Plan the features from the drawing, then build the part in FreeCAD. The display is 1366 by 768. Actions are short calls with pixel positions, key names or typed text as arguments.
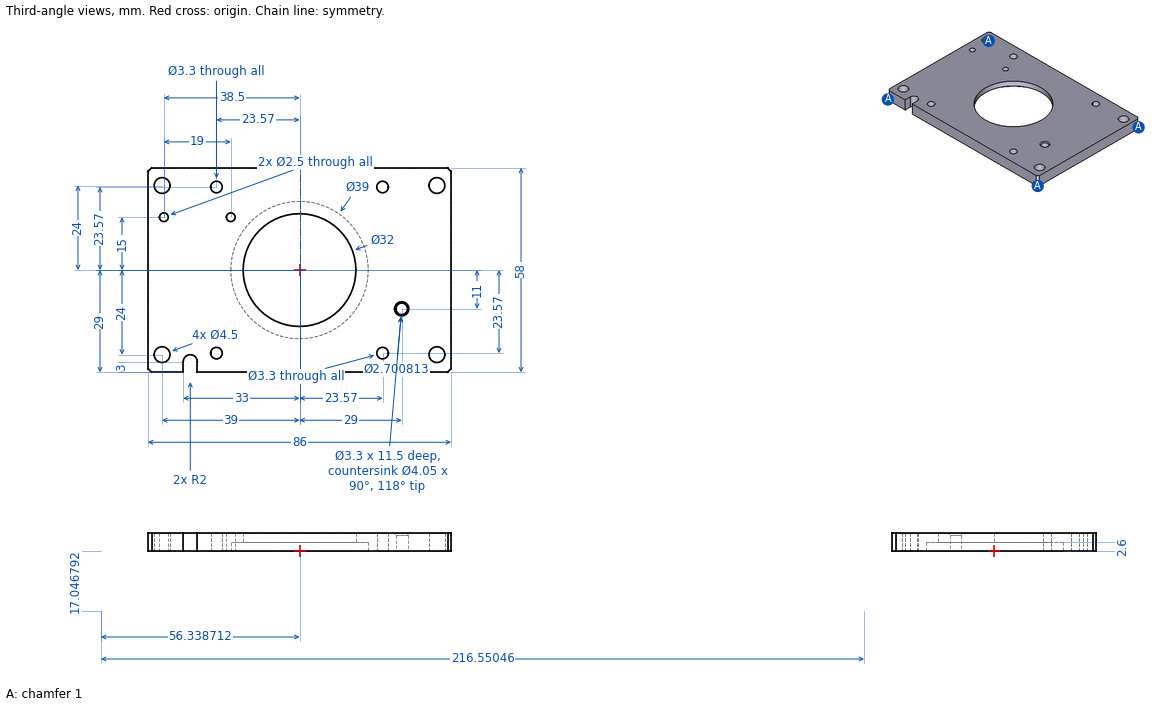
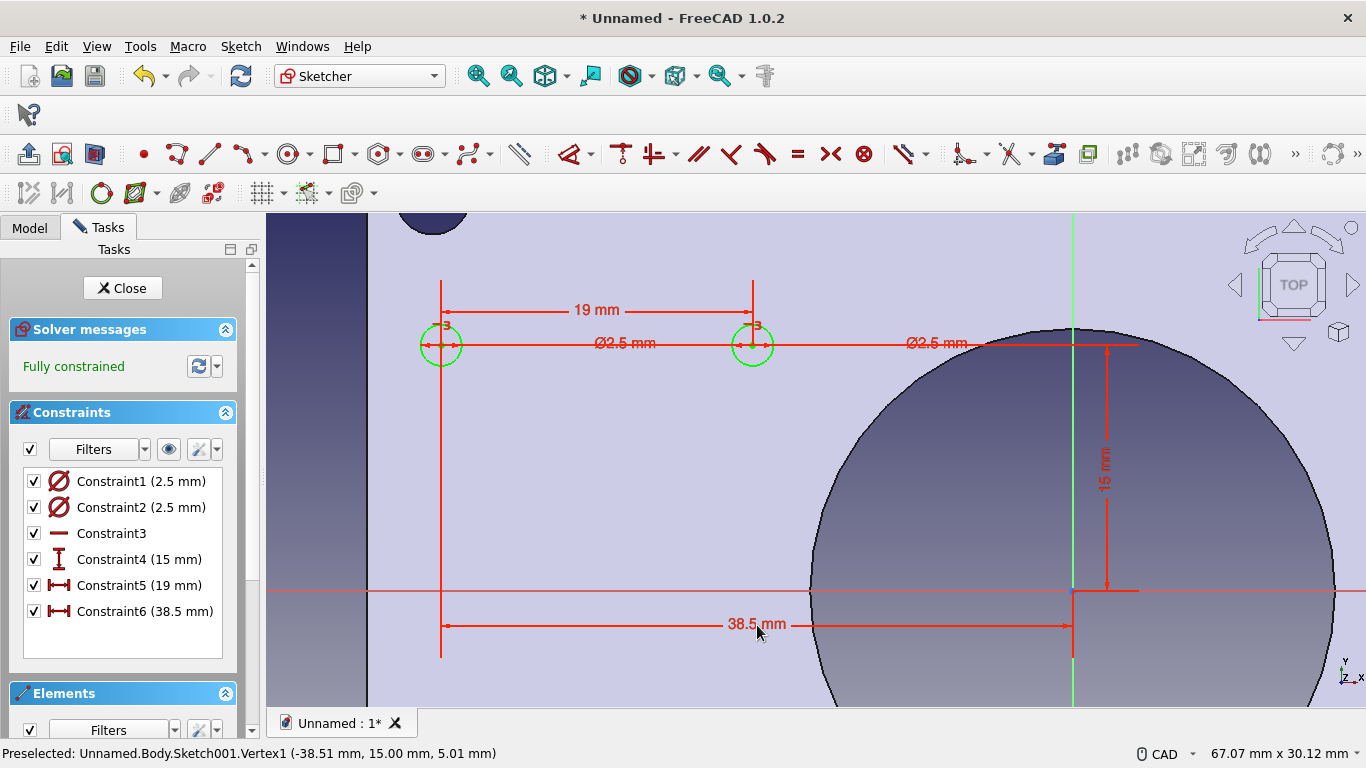
click(123, 288)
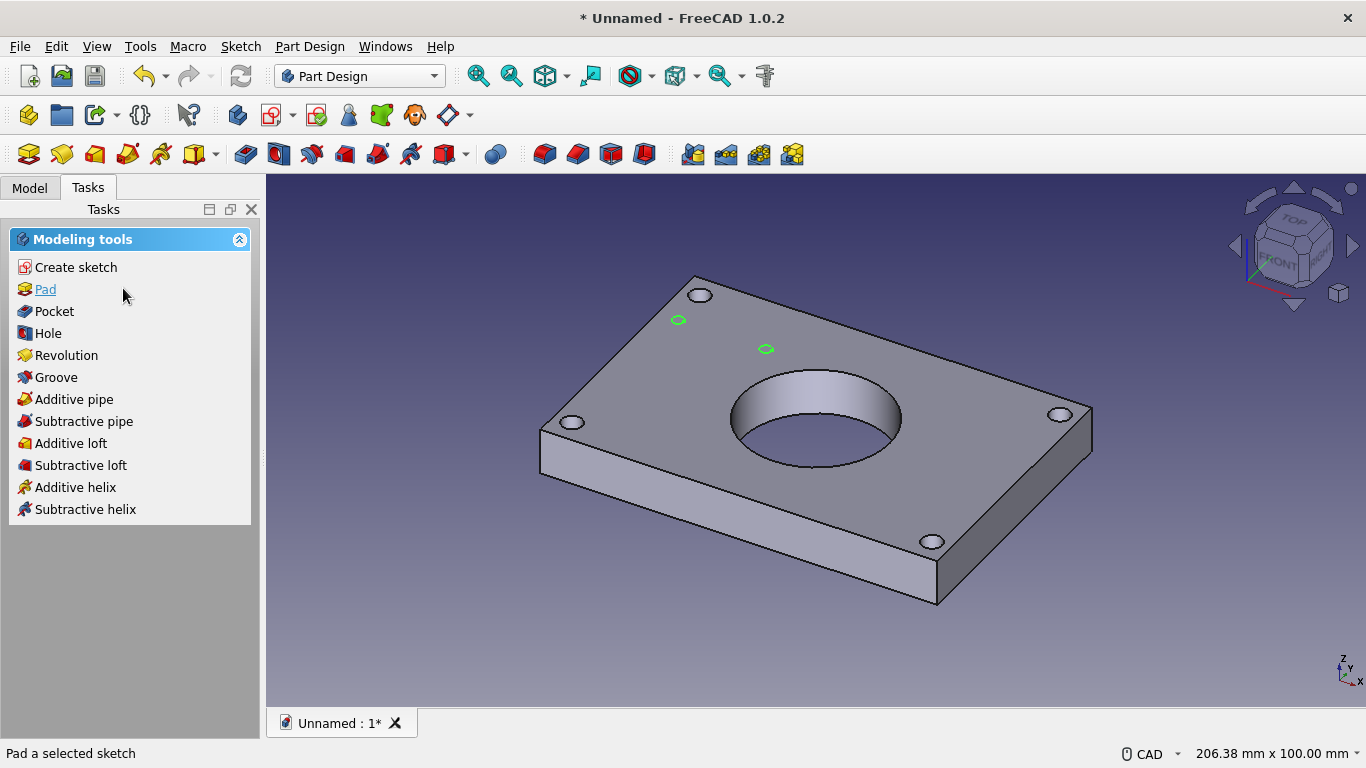
click(279, 154)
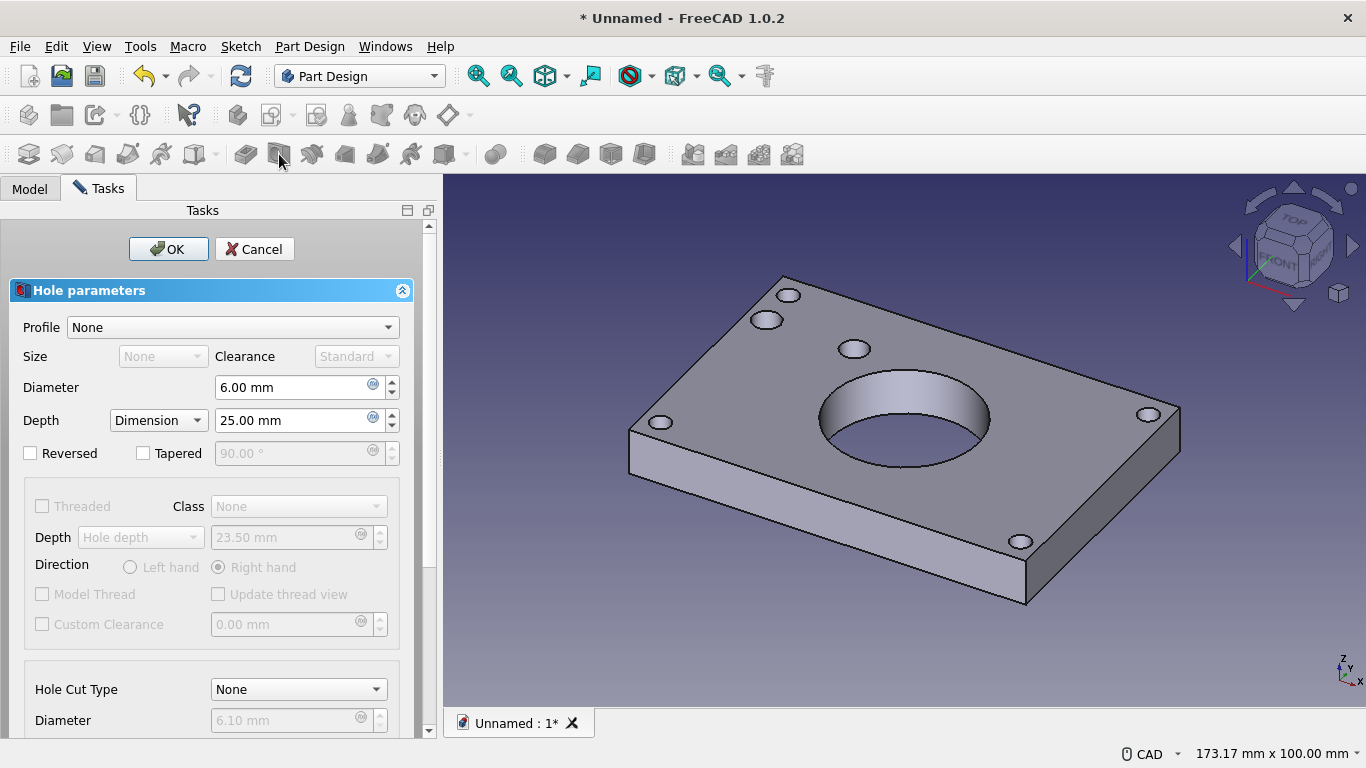
triple_click(300, 388)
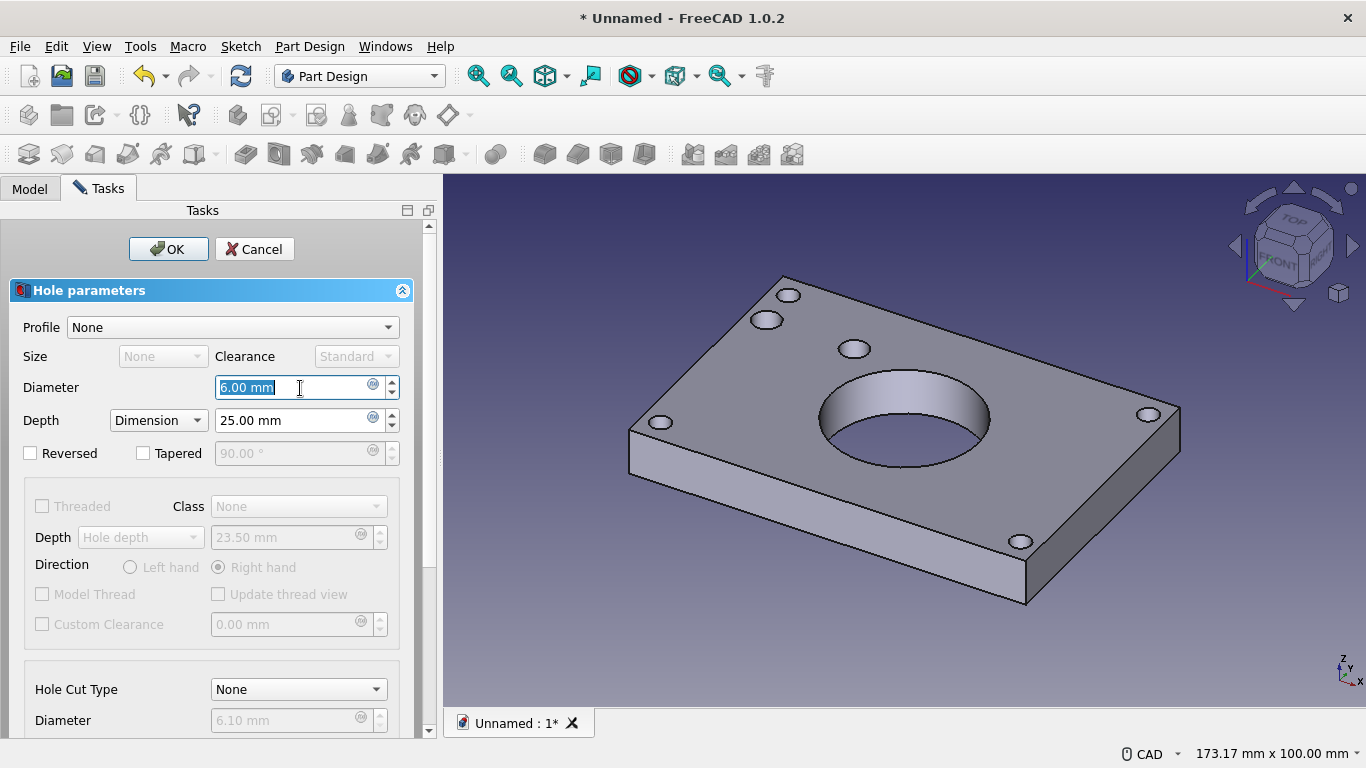
text(2.5)
key(Tab)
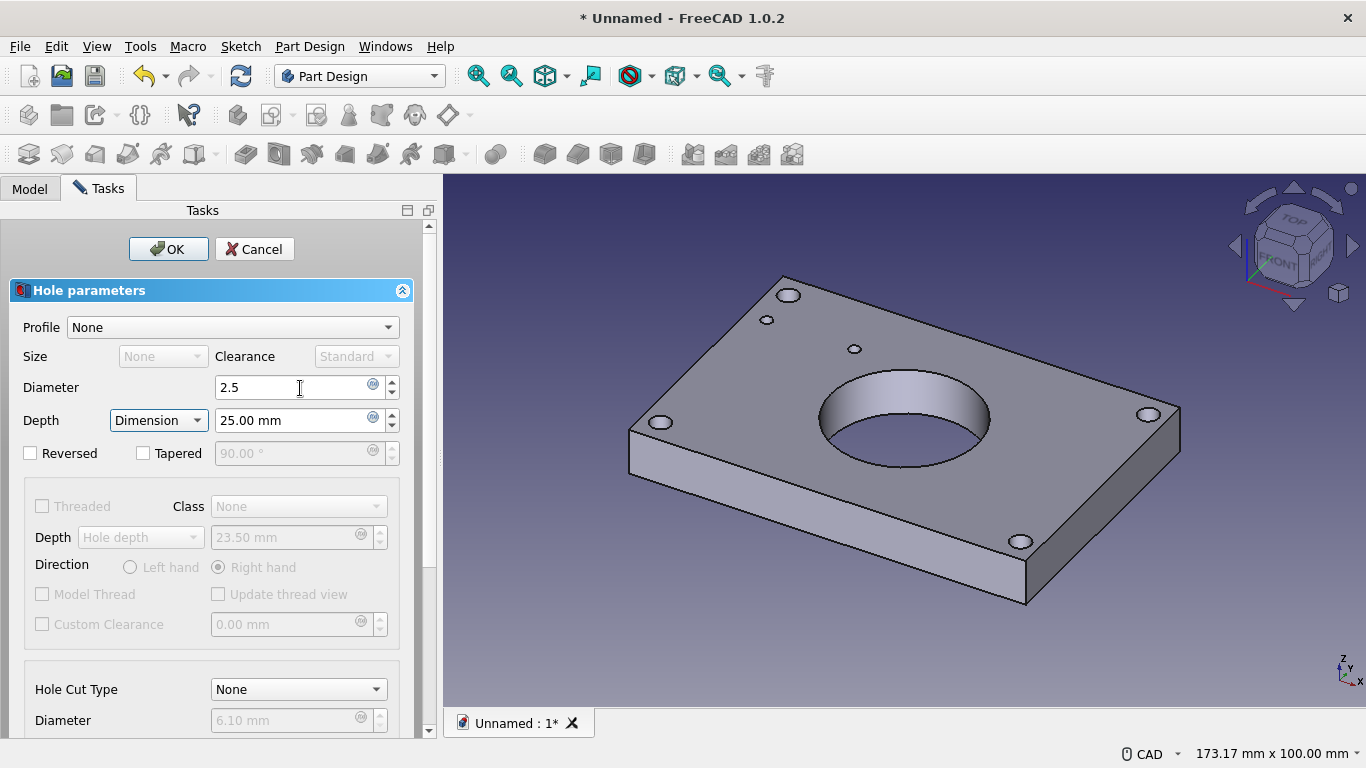
click(160, 420)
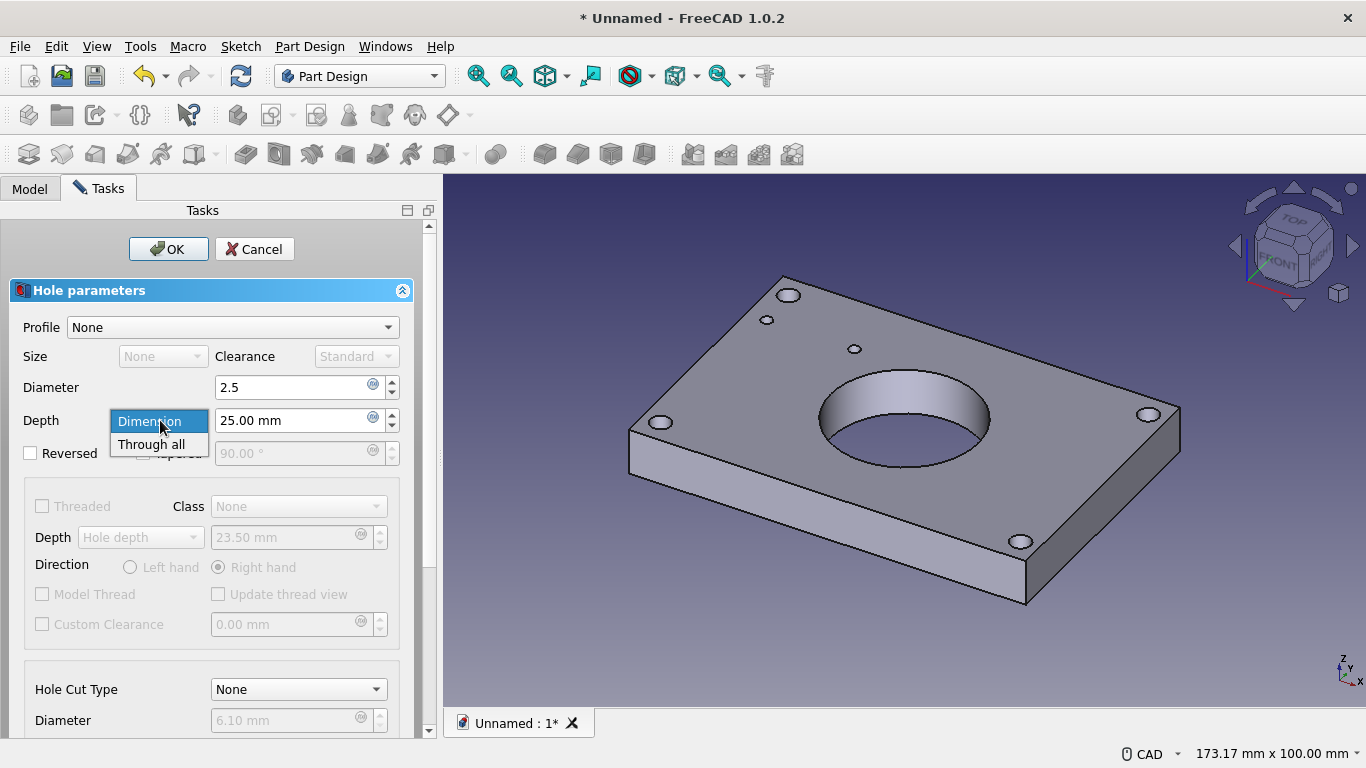
click(158, 444)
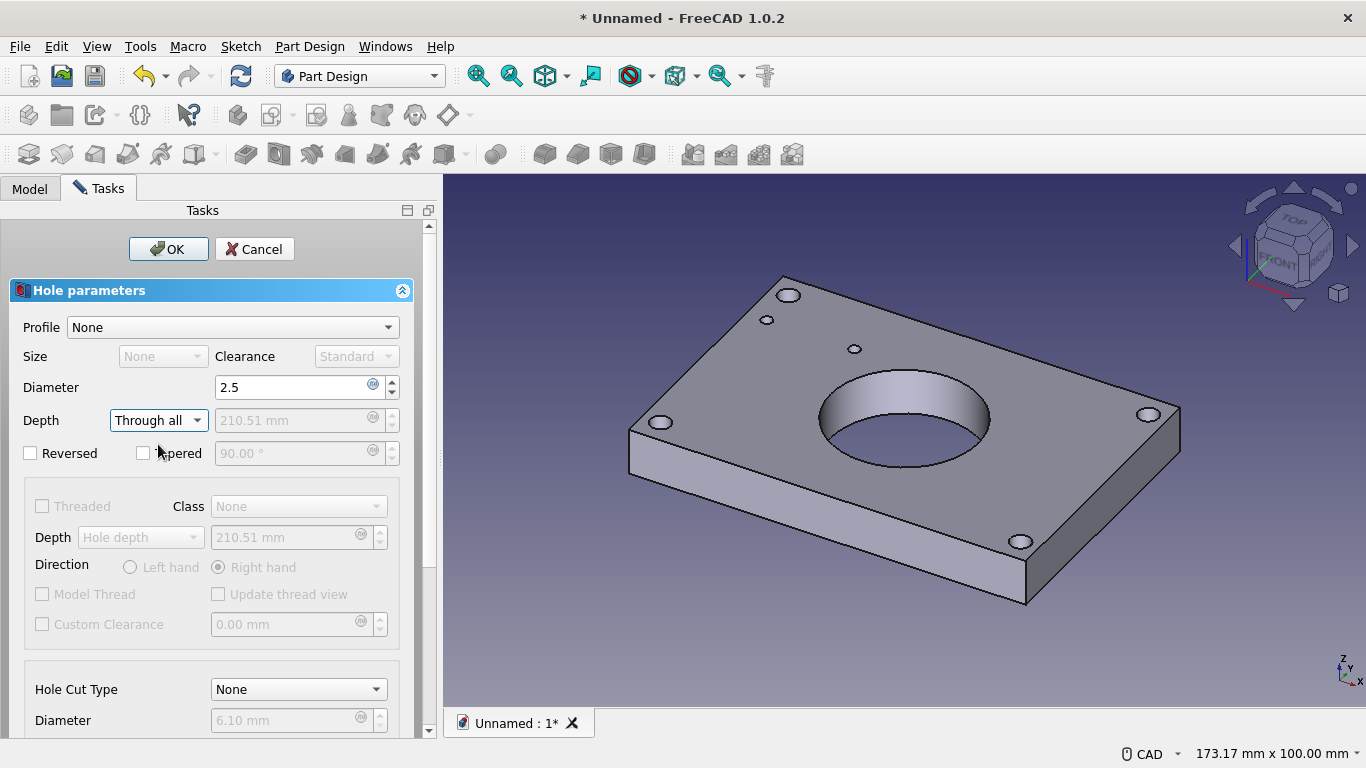
click(169, 249)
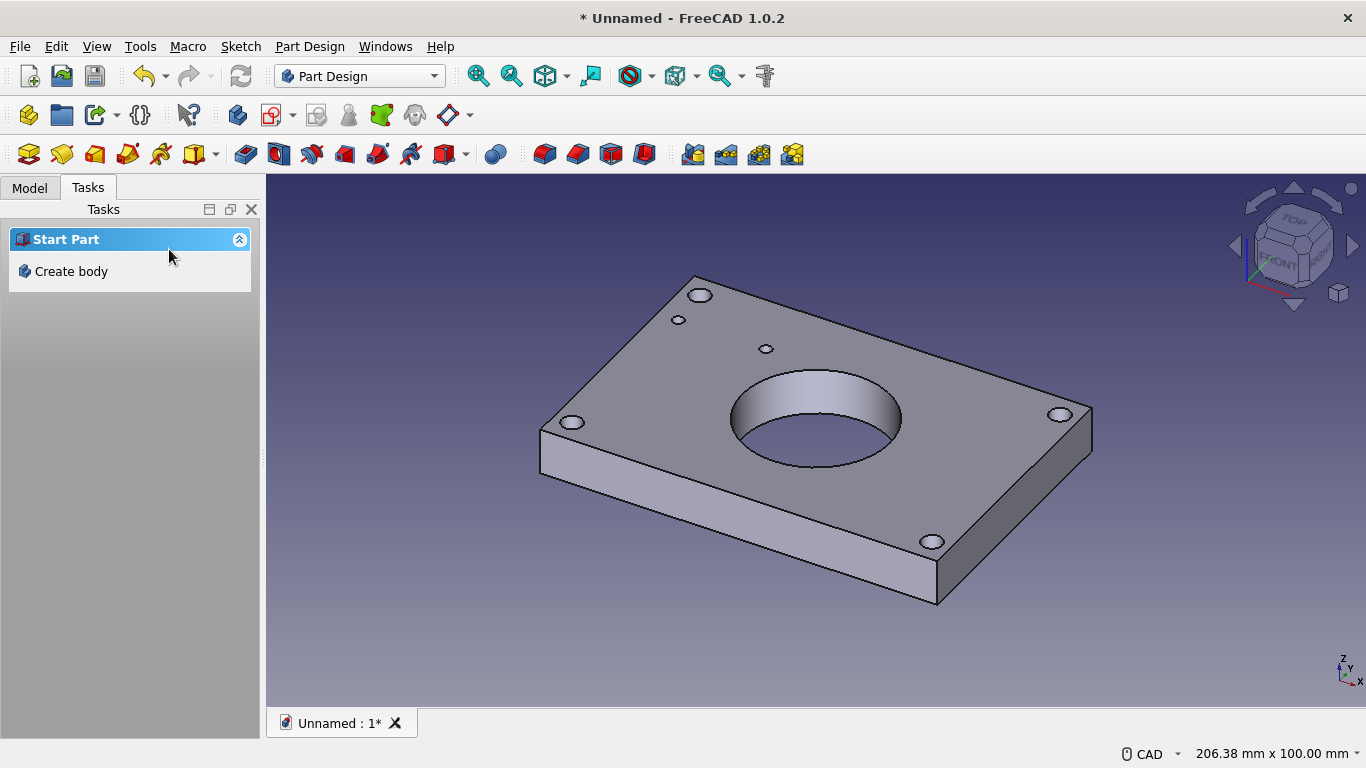
click(974, 411)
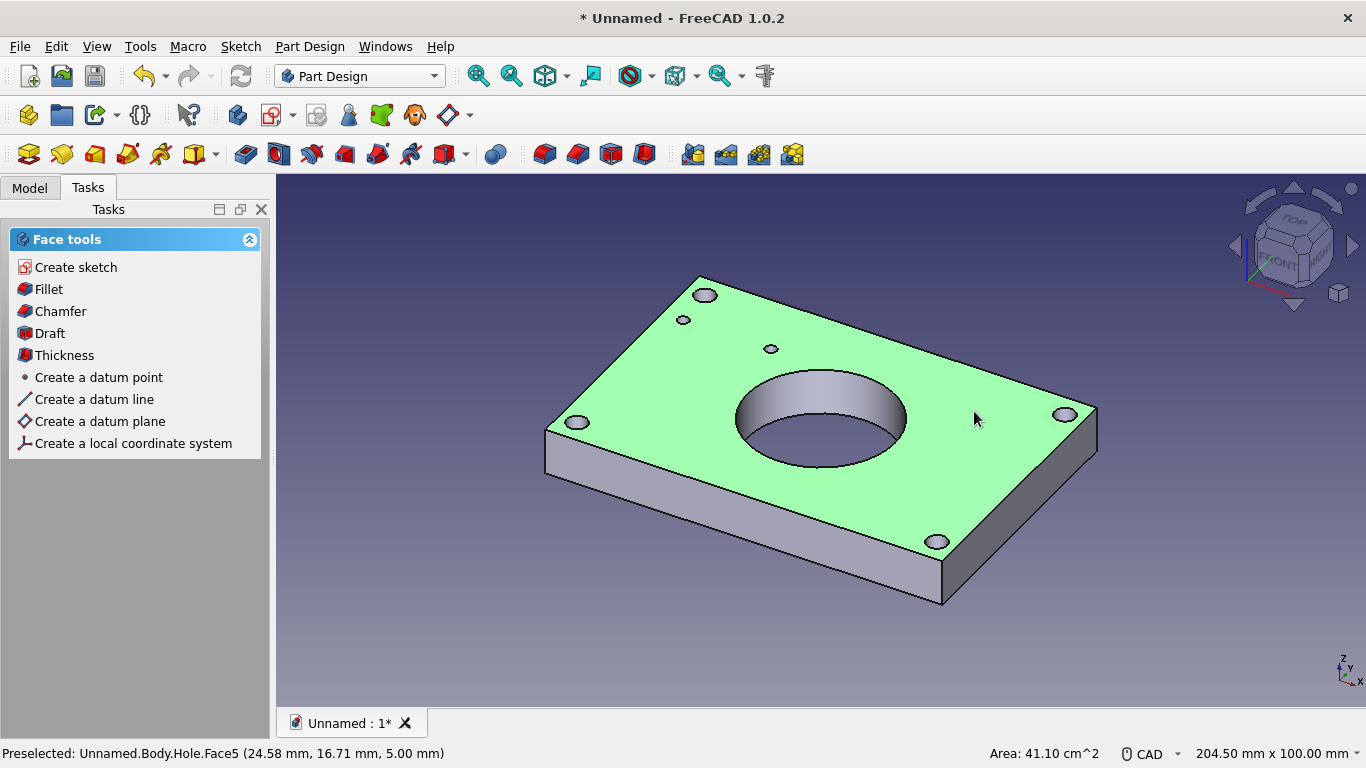
click(270, 116)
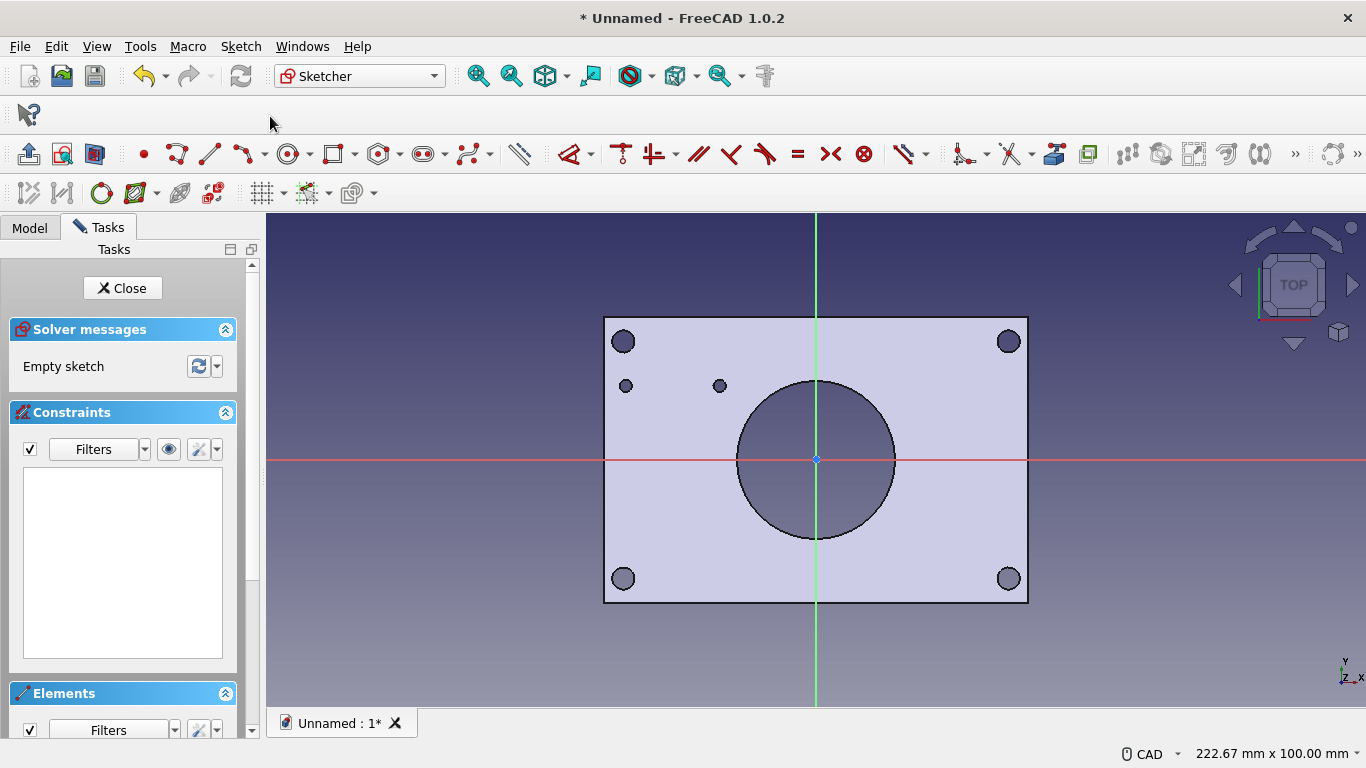
scroll(697, 337, up, 15)